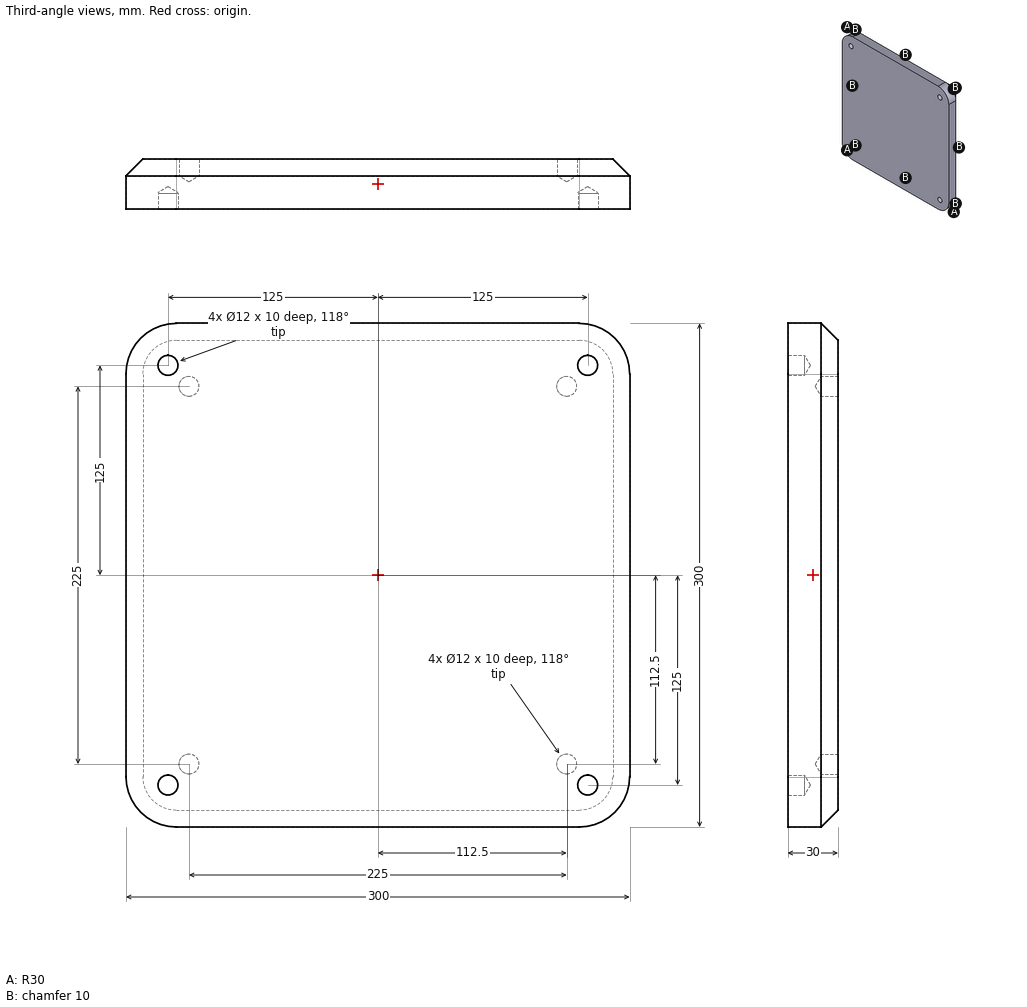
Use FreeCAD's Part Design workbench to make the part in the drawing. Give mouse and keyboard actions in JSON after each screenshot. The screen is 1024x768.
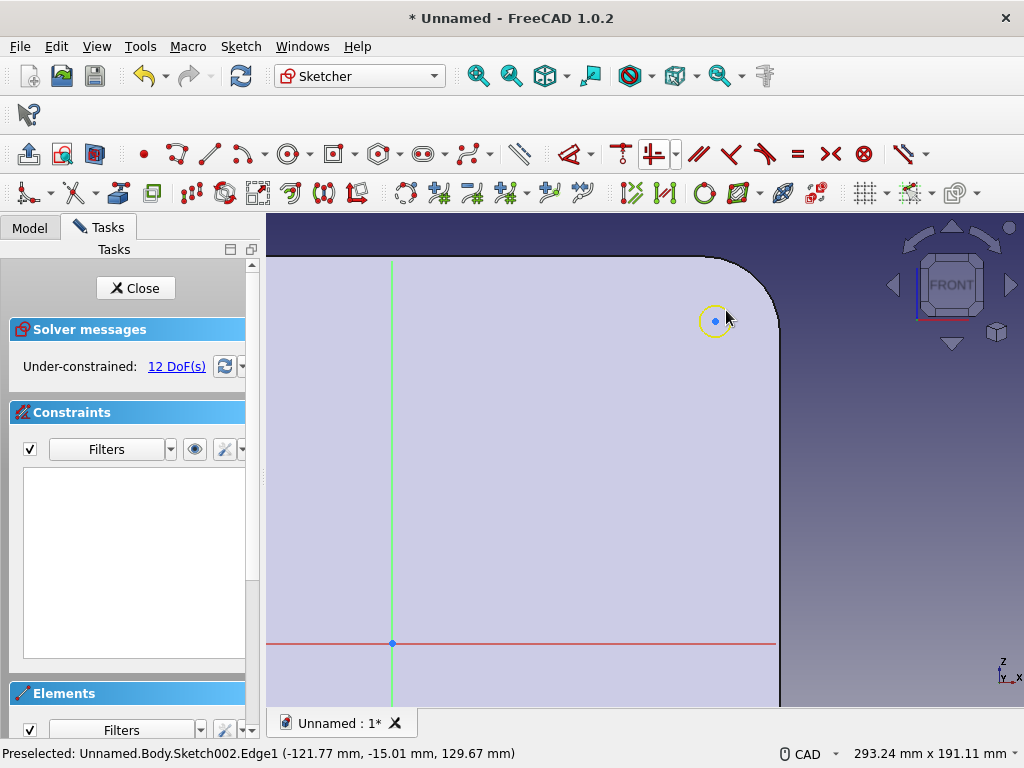
{"action": "left_click", "coordinate": [726, 310]}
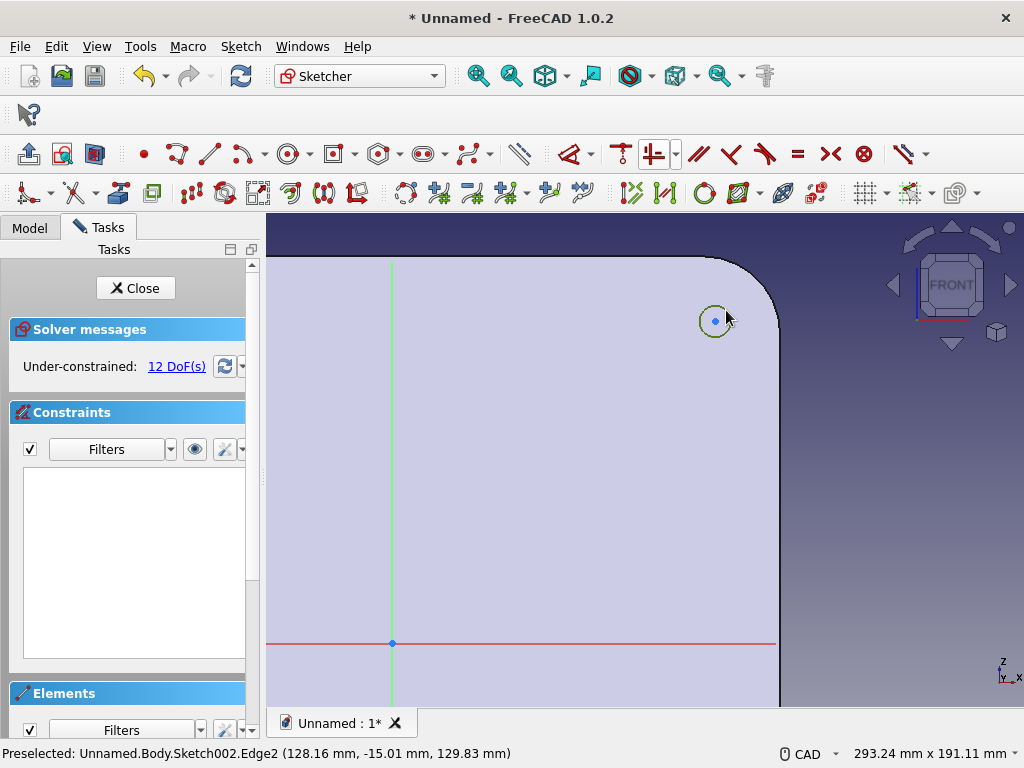
{"action": "scroll", "coordinate": [727, 310], "scroll_direction": "down", "scroll_amount": 4}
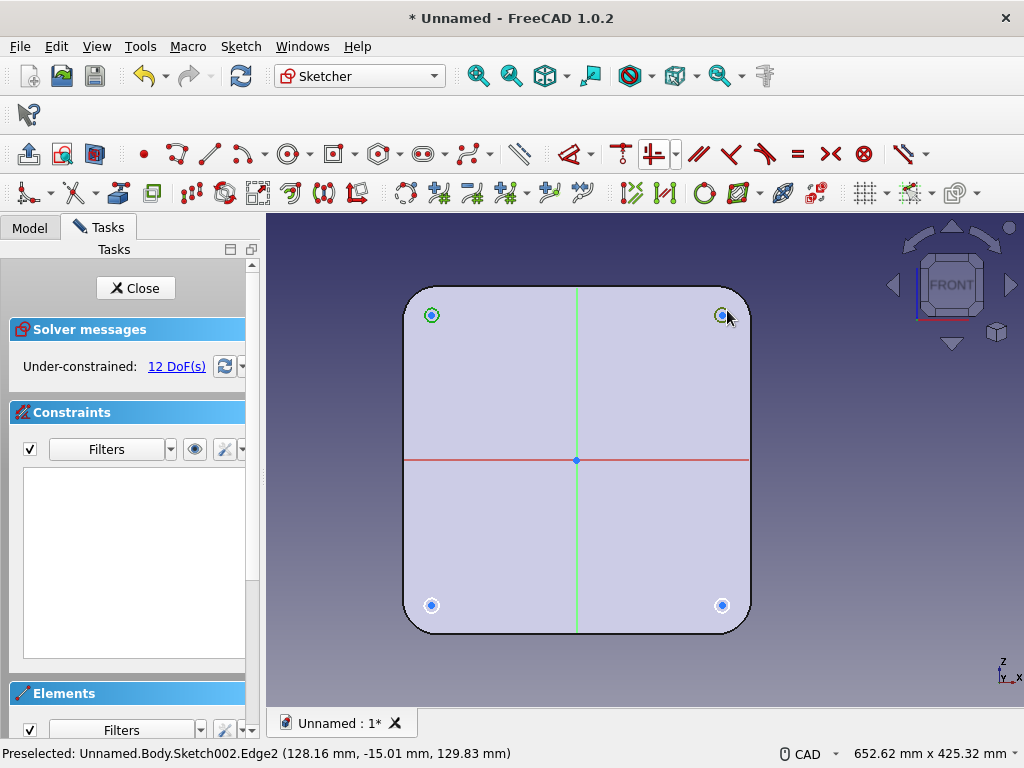
{"action": "scroll", "coordinate": [727, 601], "scroll_direction": "up", "scroll_amount": 4}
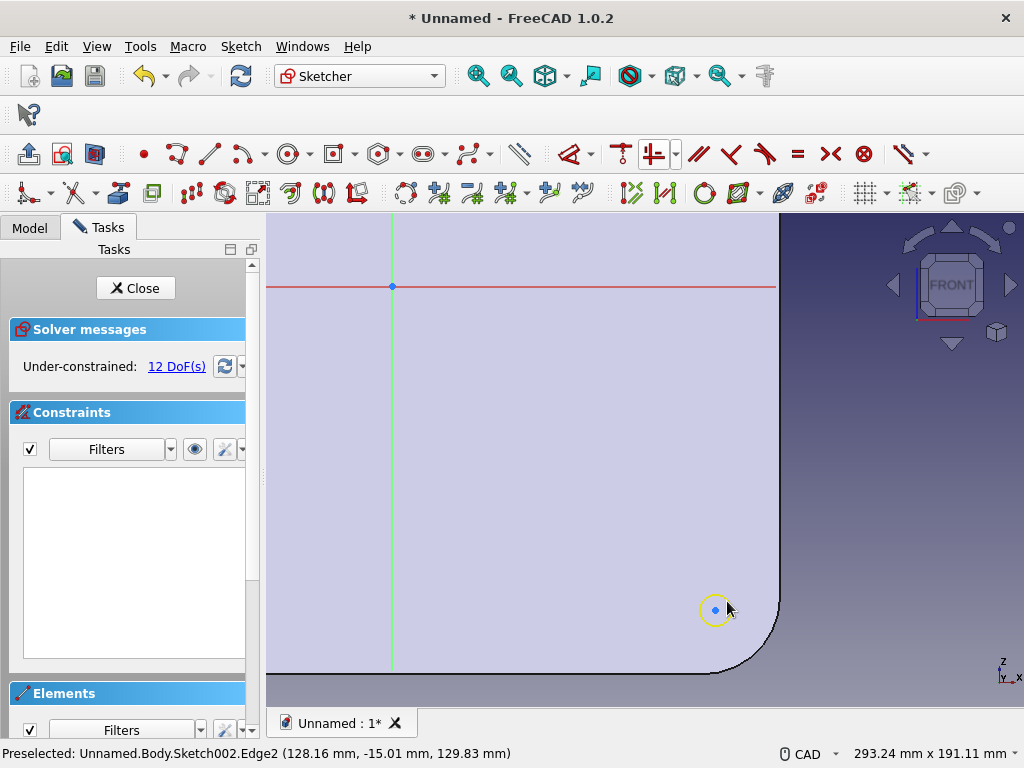
{"action": "left_click", "coordinate": [727, 599]}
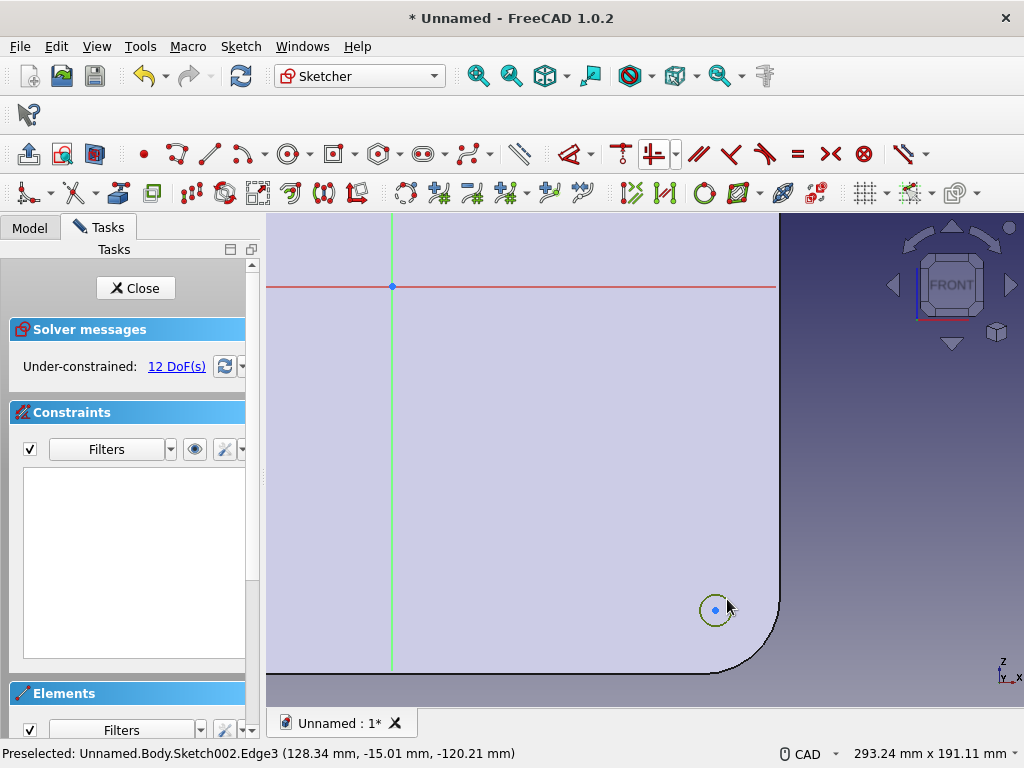
{"action": "scroll", "coordinate": [727, 602], "scroll_direction": "down", "scroll_amount": 4}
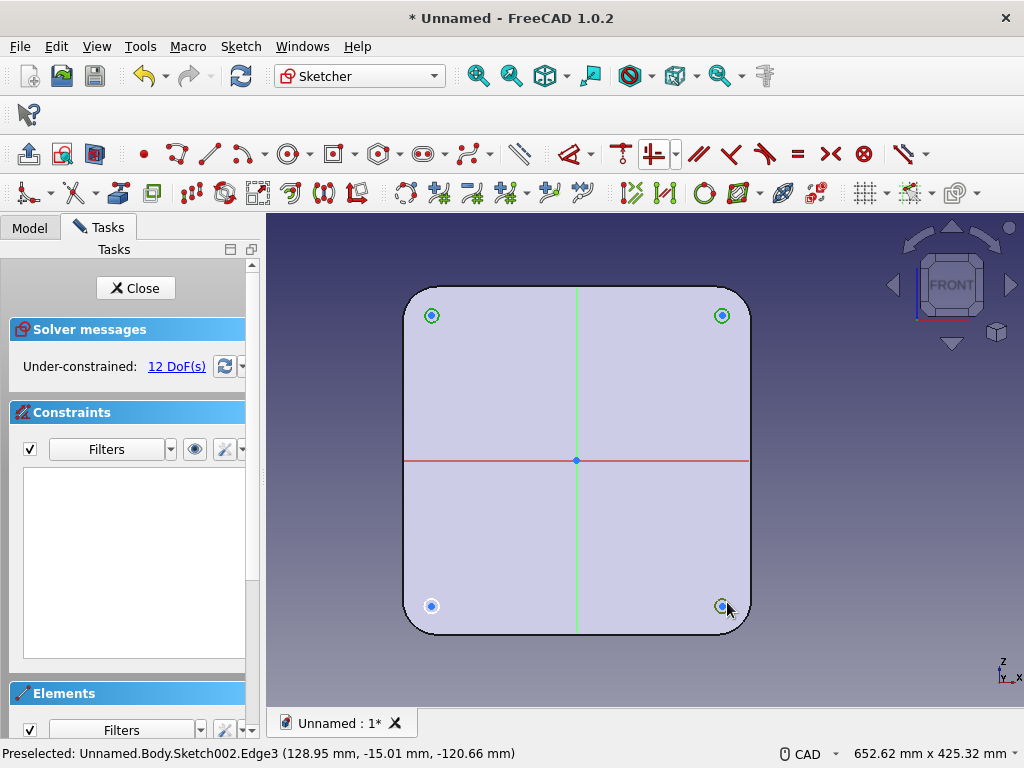
{"action": "scroll", "coordinate": [437, 601], "scroll_direction": "up", "scroll_amount": 4}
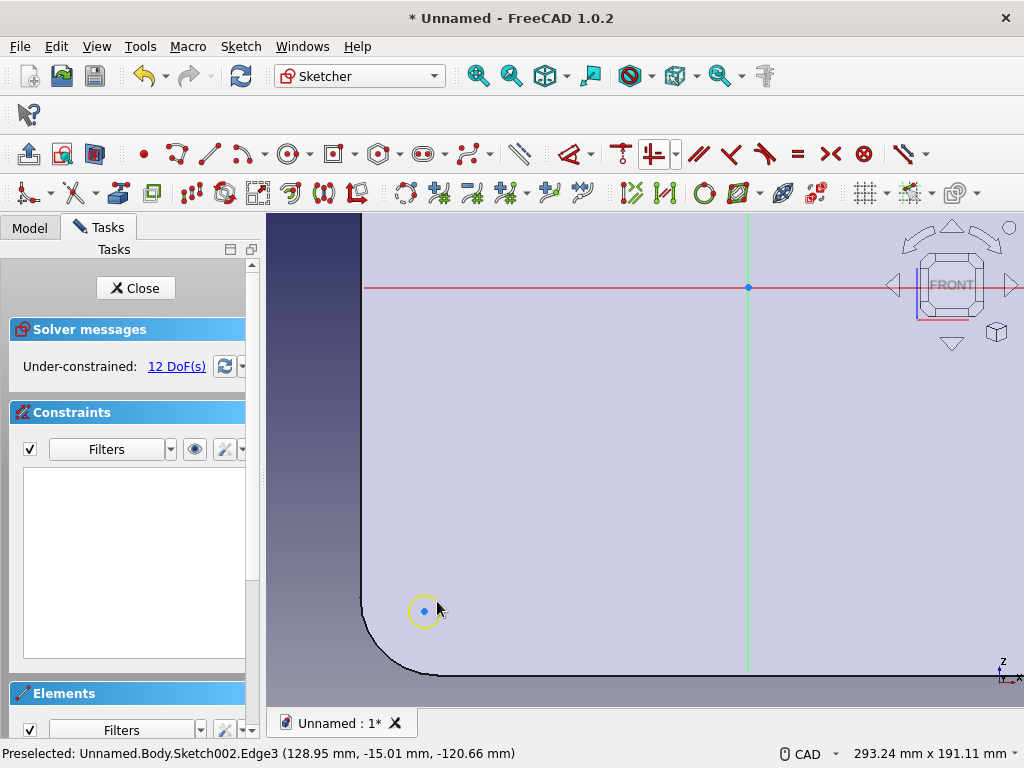
{"action": "left_click", "coordinate": [436, 600]}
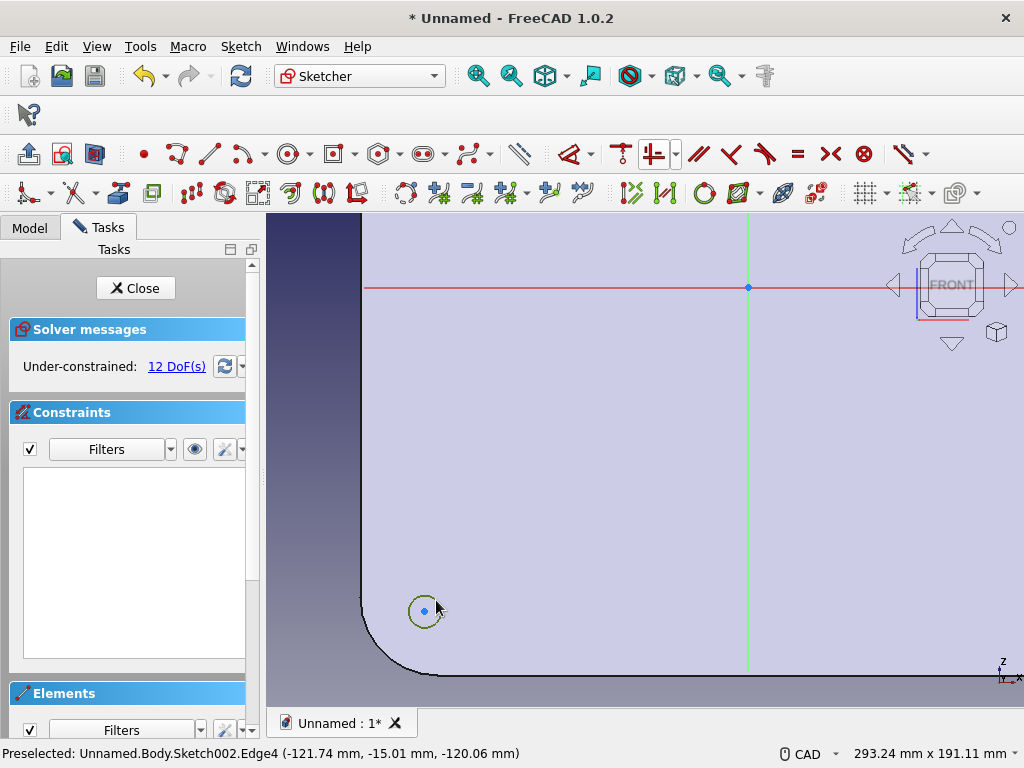
{"action": "left_click", "coordinate": [798, 154]}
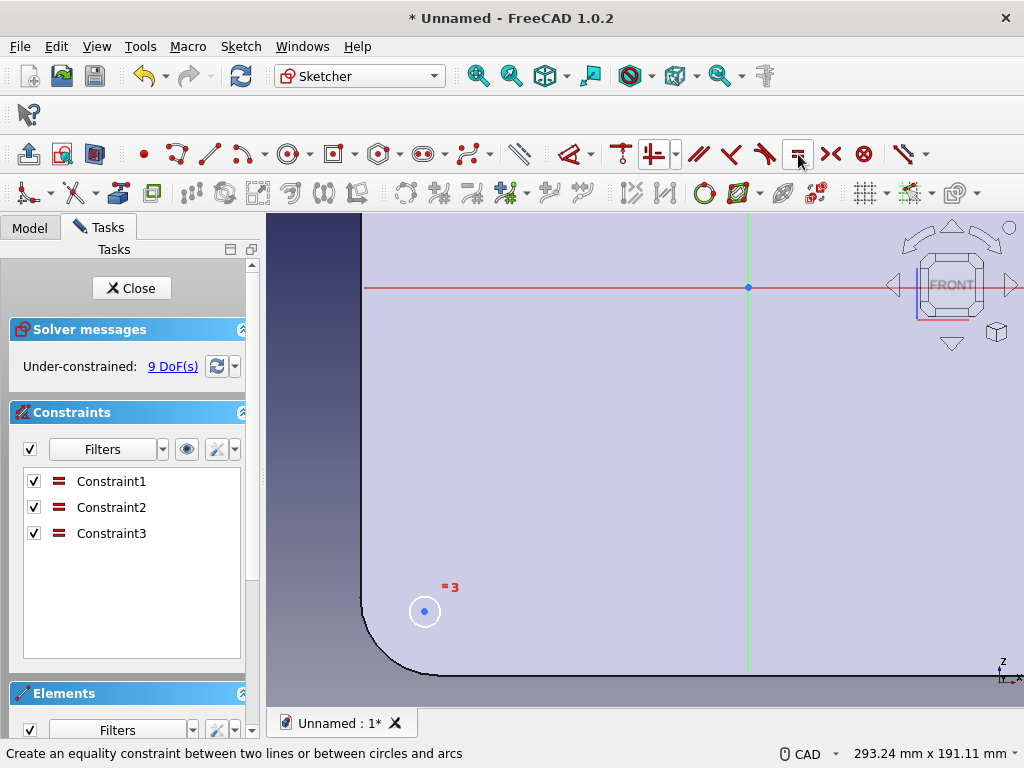
{"action": "left_click", "coordinate": [568, 154]}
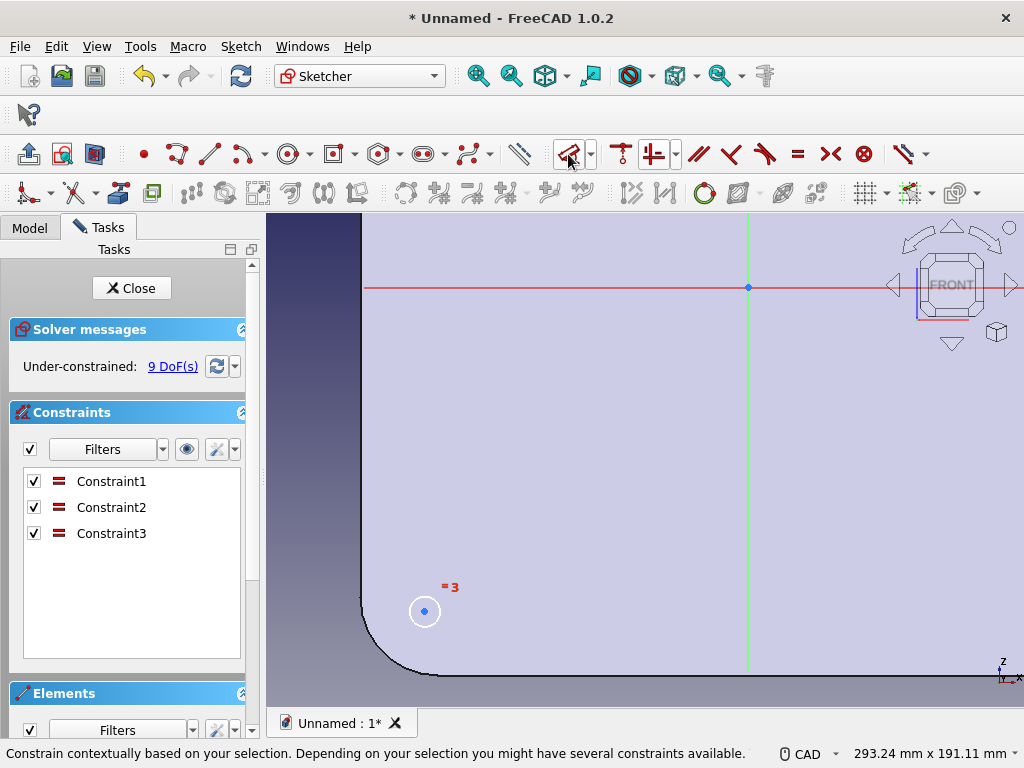
{"action": "scroll", "coordinate": [436, 601], "scroll_direction": "down", "scroll_amount": 4}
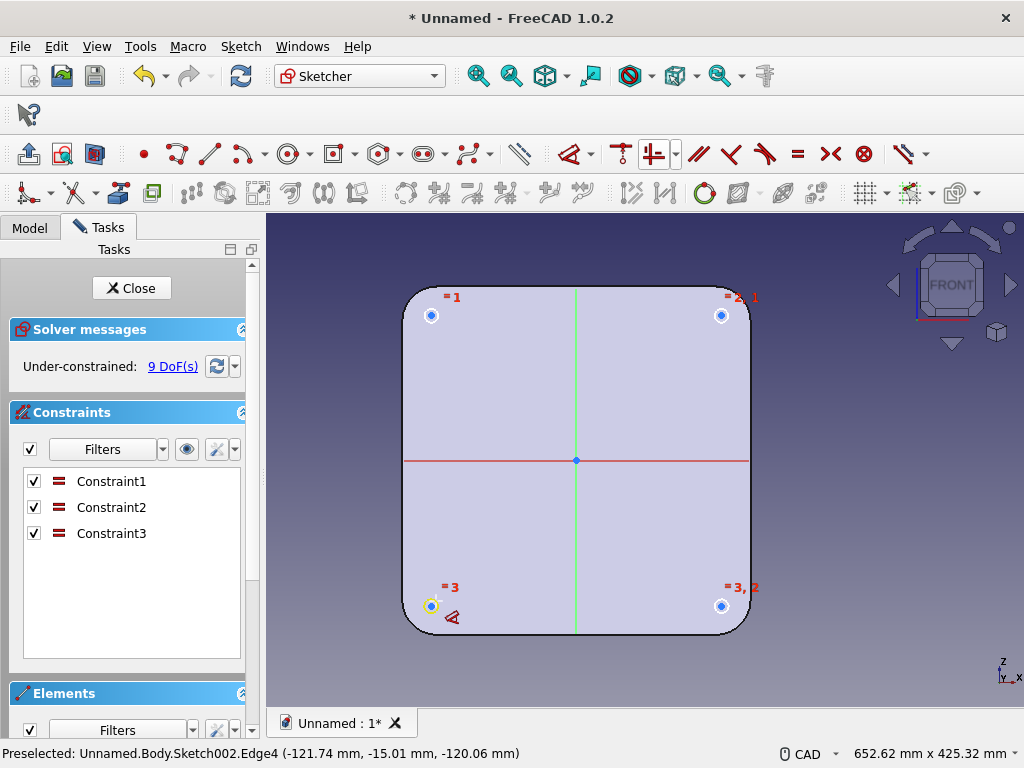
{"action": "scroll", "coordinate": [436, 311], "scroll_direction": "up", "scroll_amount": 6}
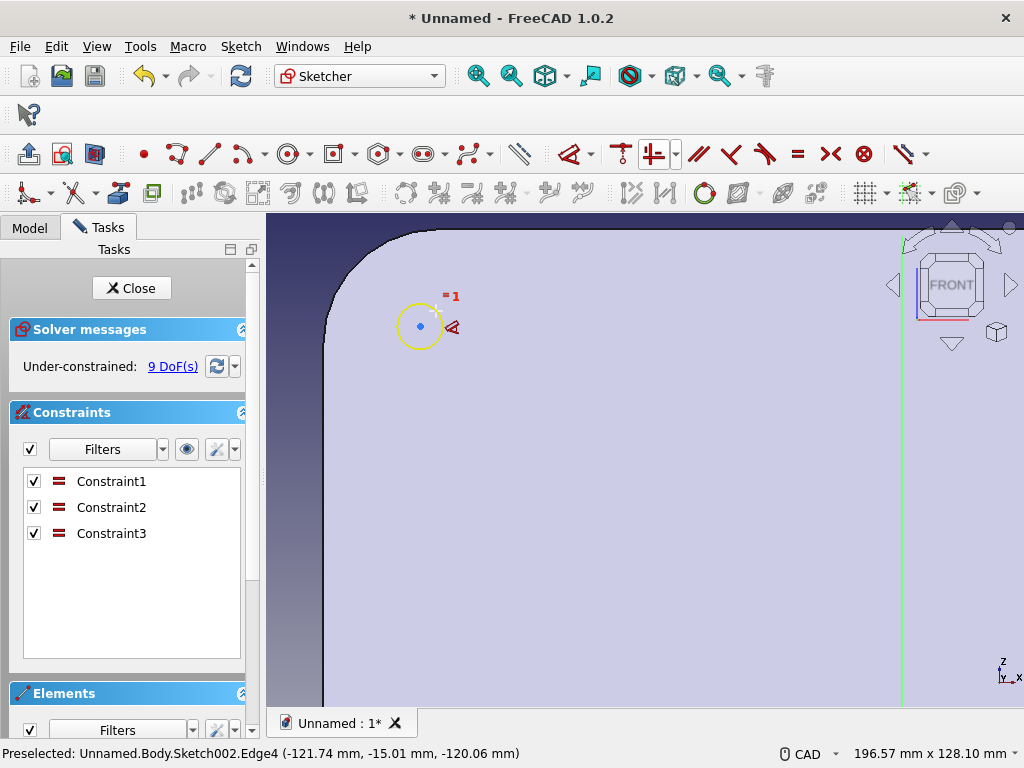
{"action": "left_click", "coordinate": [436, 311]}
{"action": "left_click", "coordinate": [459, 289]}